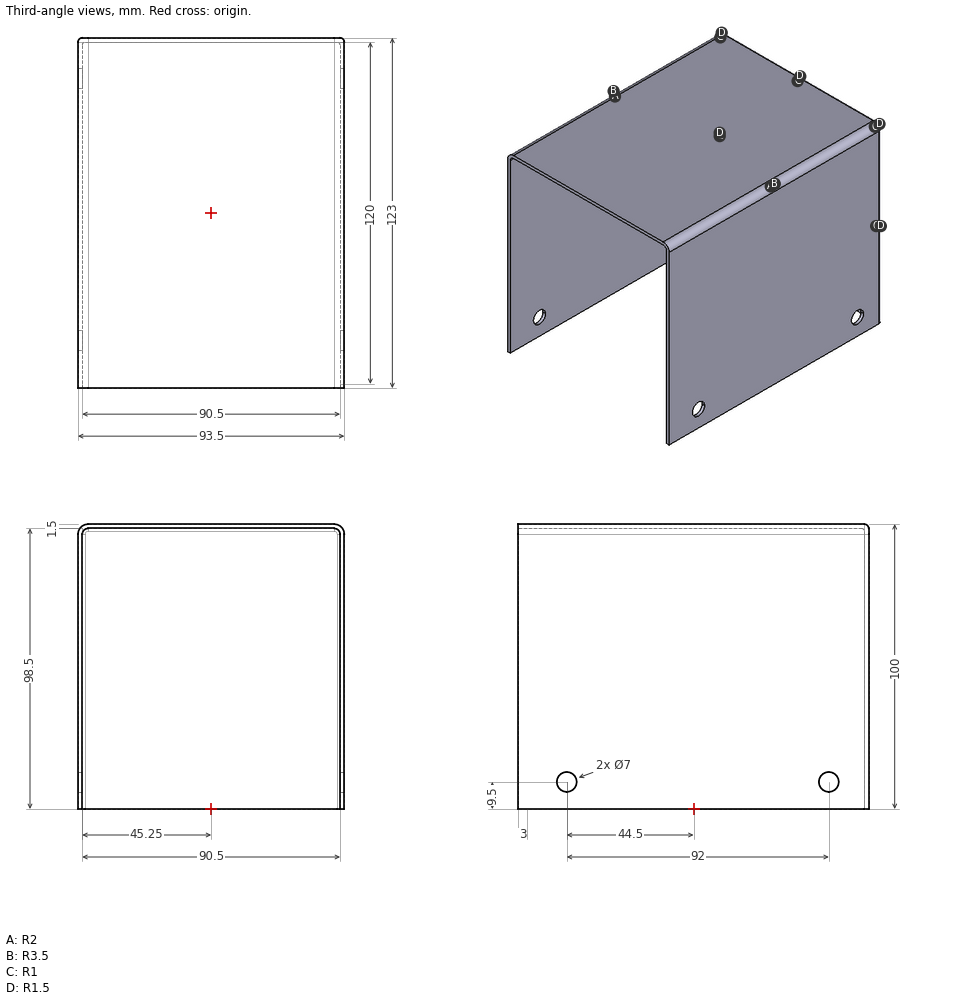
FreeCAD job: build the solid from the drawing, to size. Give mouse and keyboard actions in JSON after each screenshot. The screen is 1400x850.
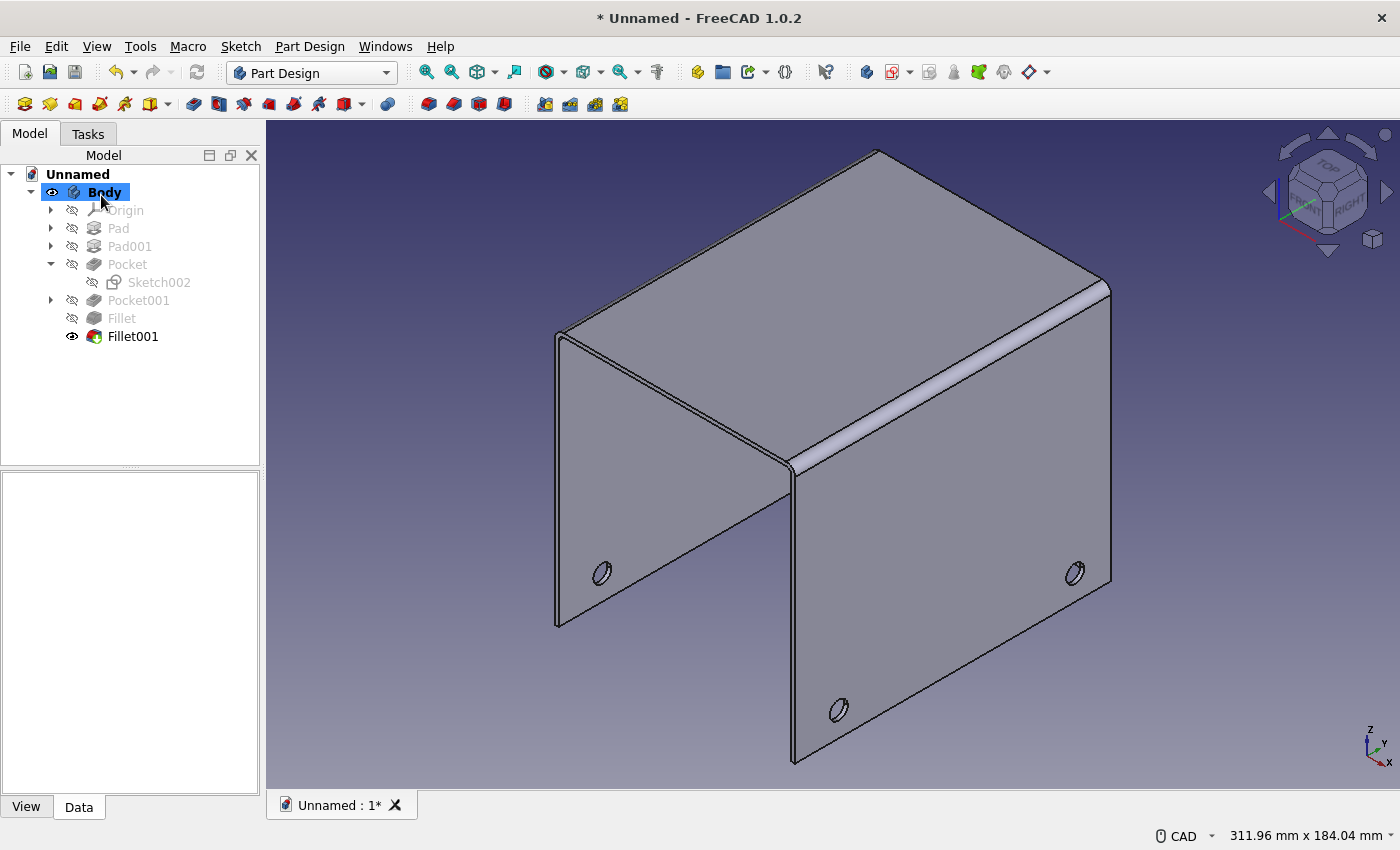
{"action": "key", "text": "2"}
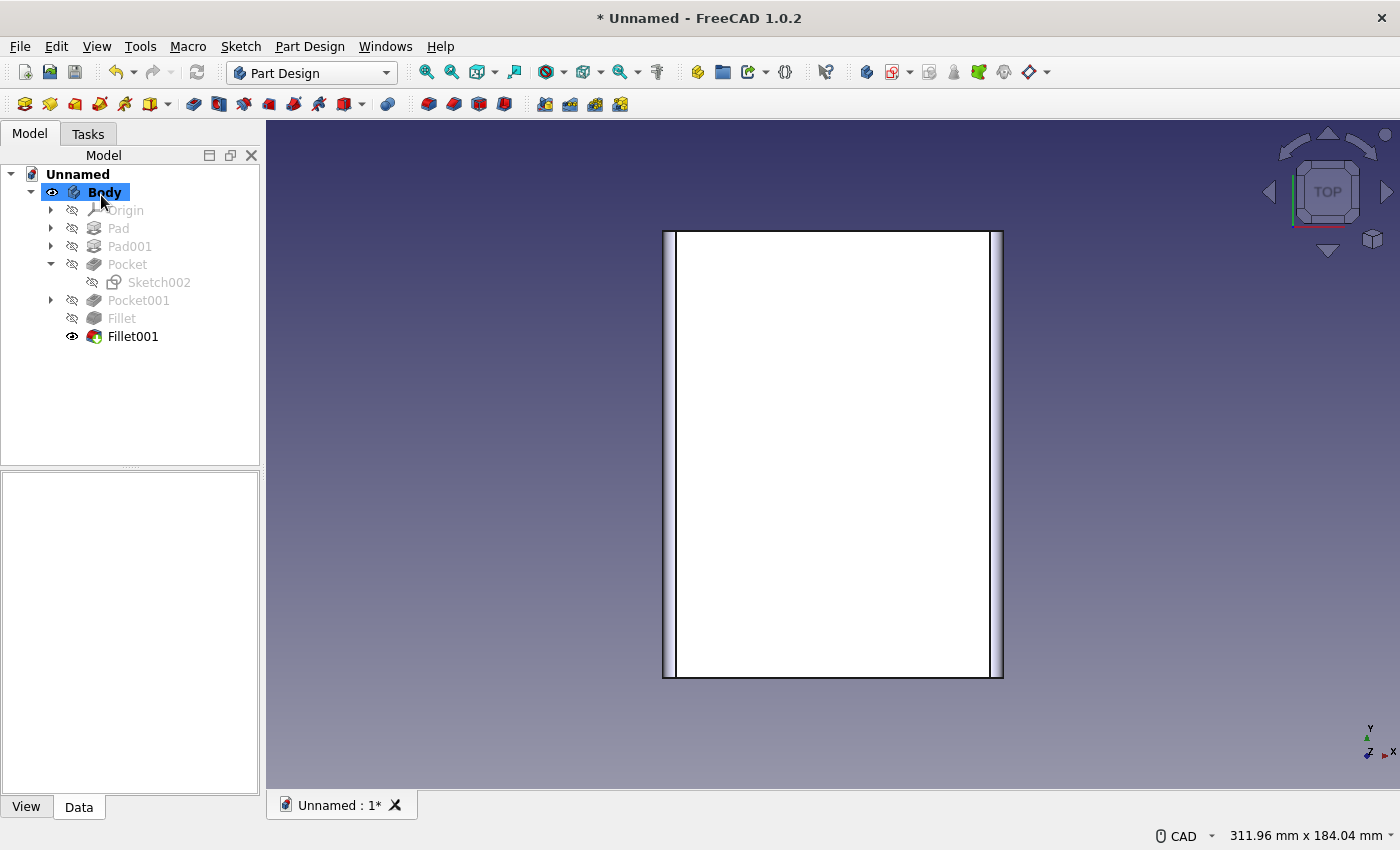
{"action": "key", "text": "1"}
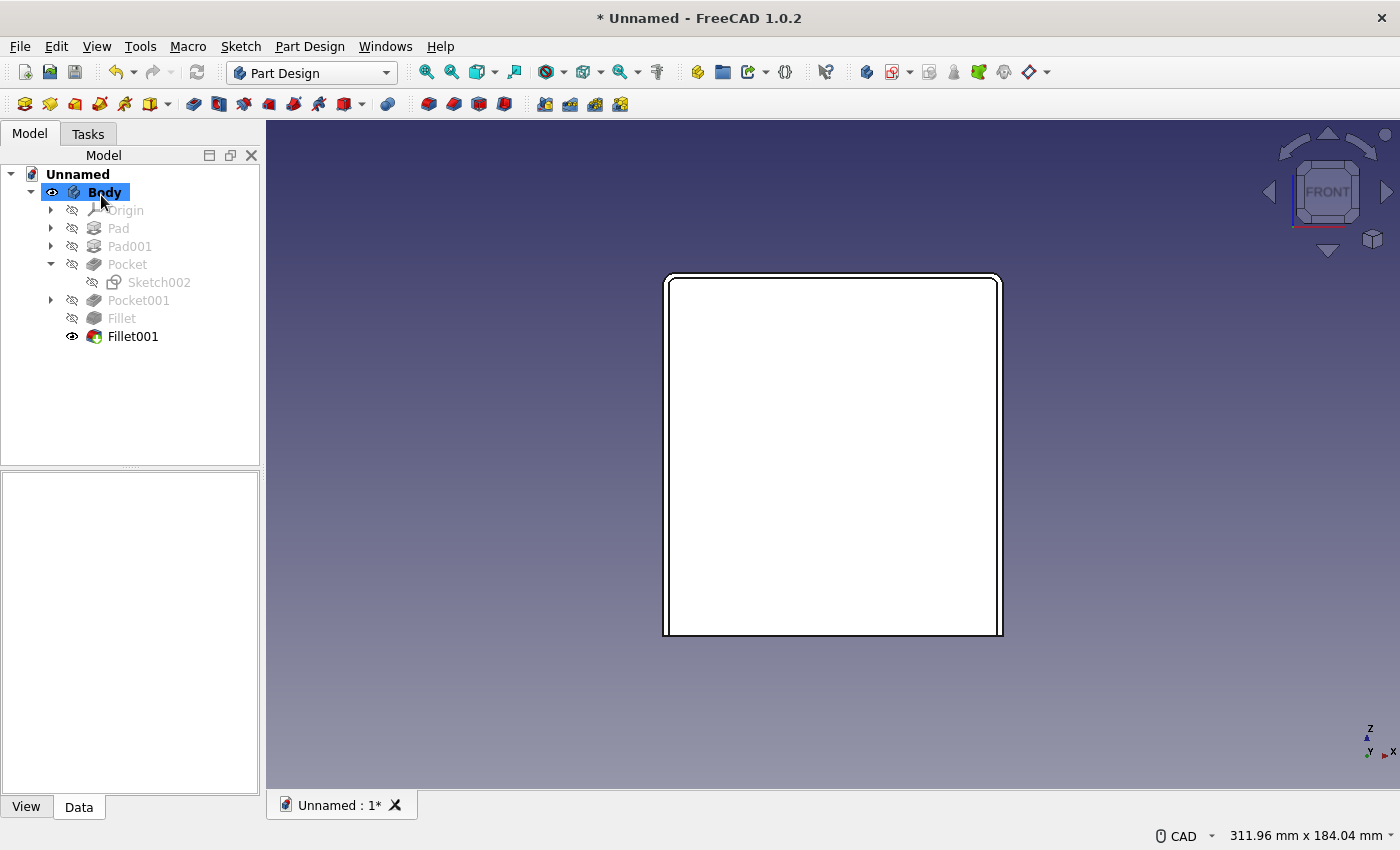
{"action": "key", "text": "3"}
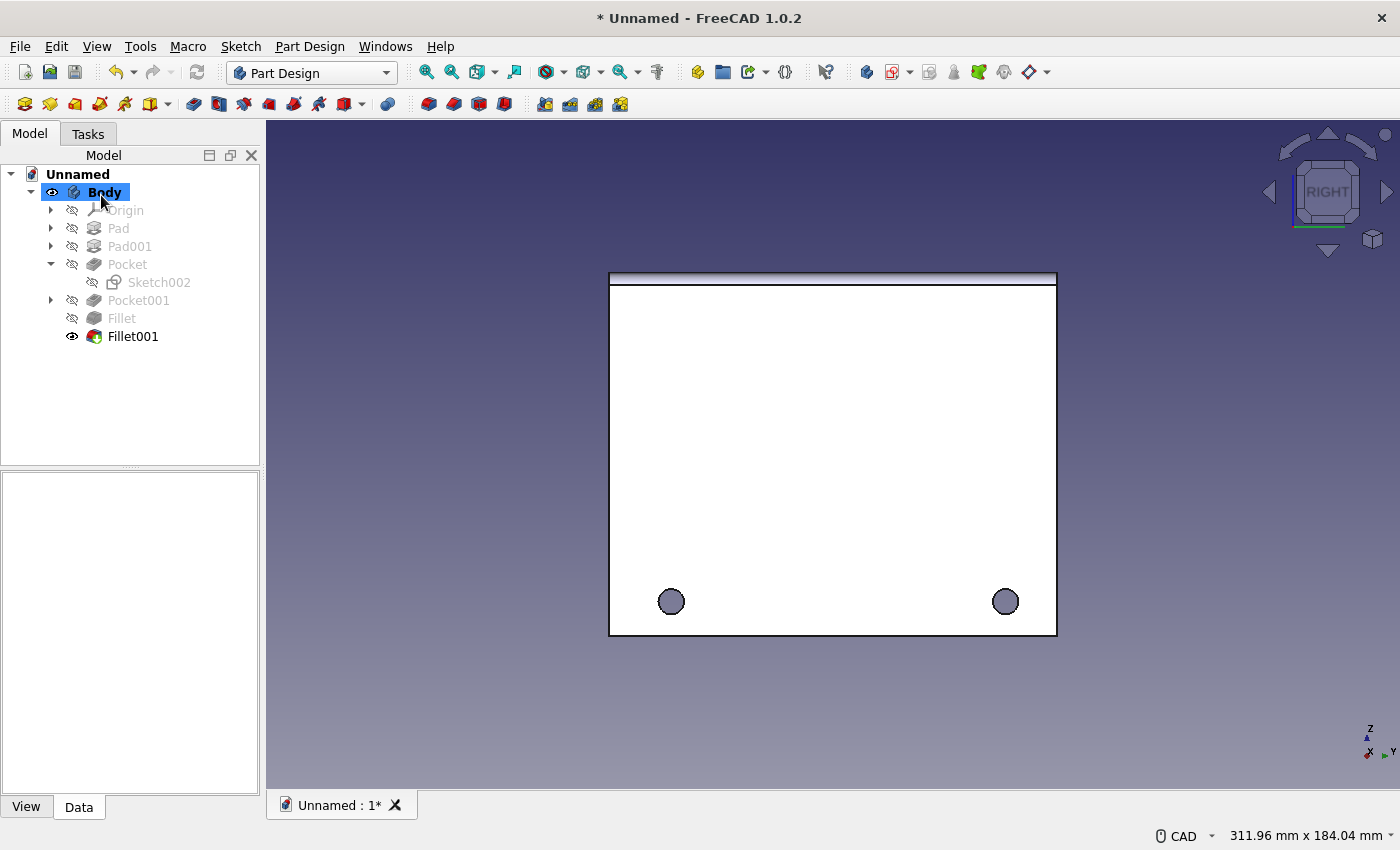
{"action": "key", "text": "5"}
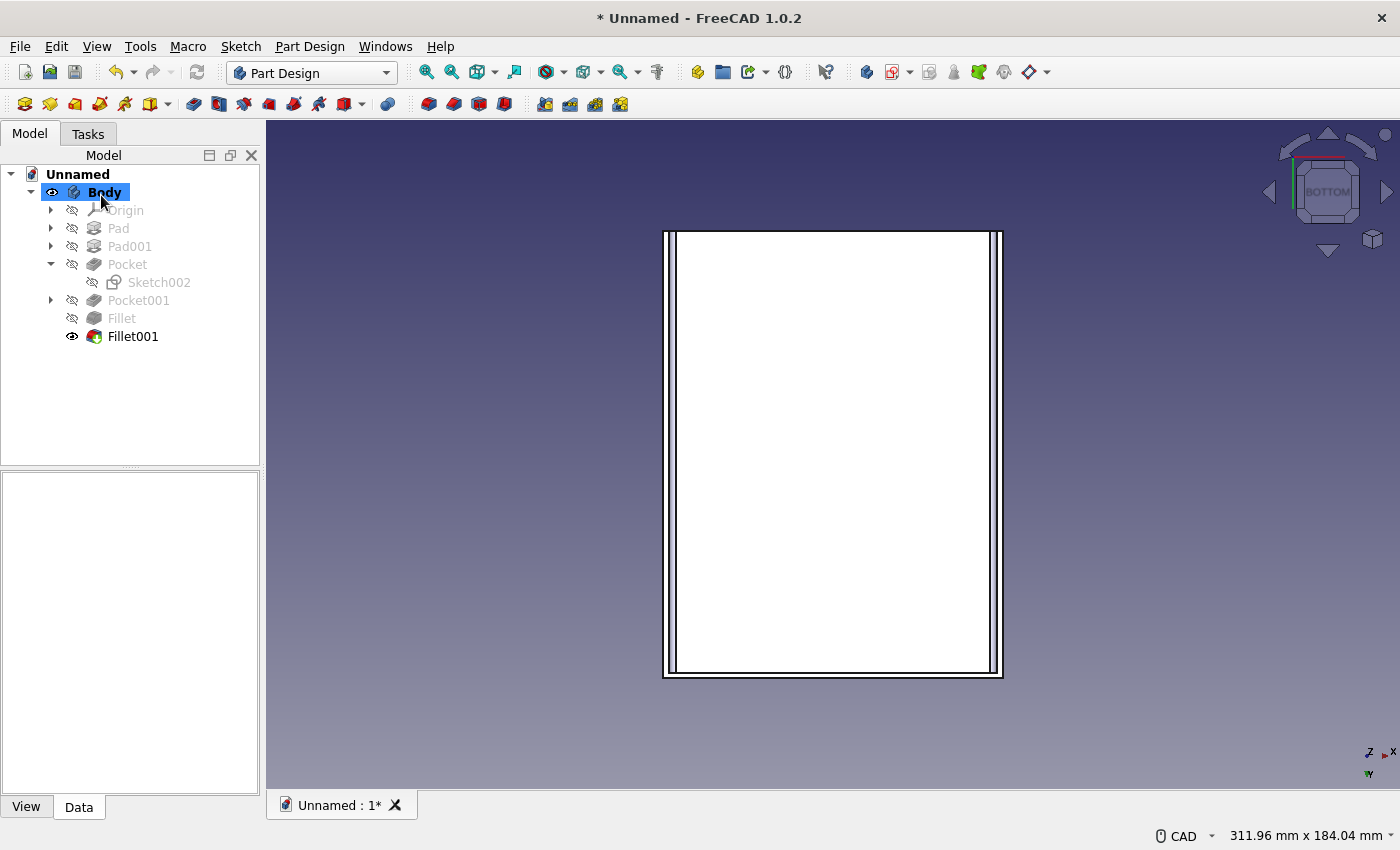
{"action": "key", "text": "4"}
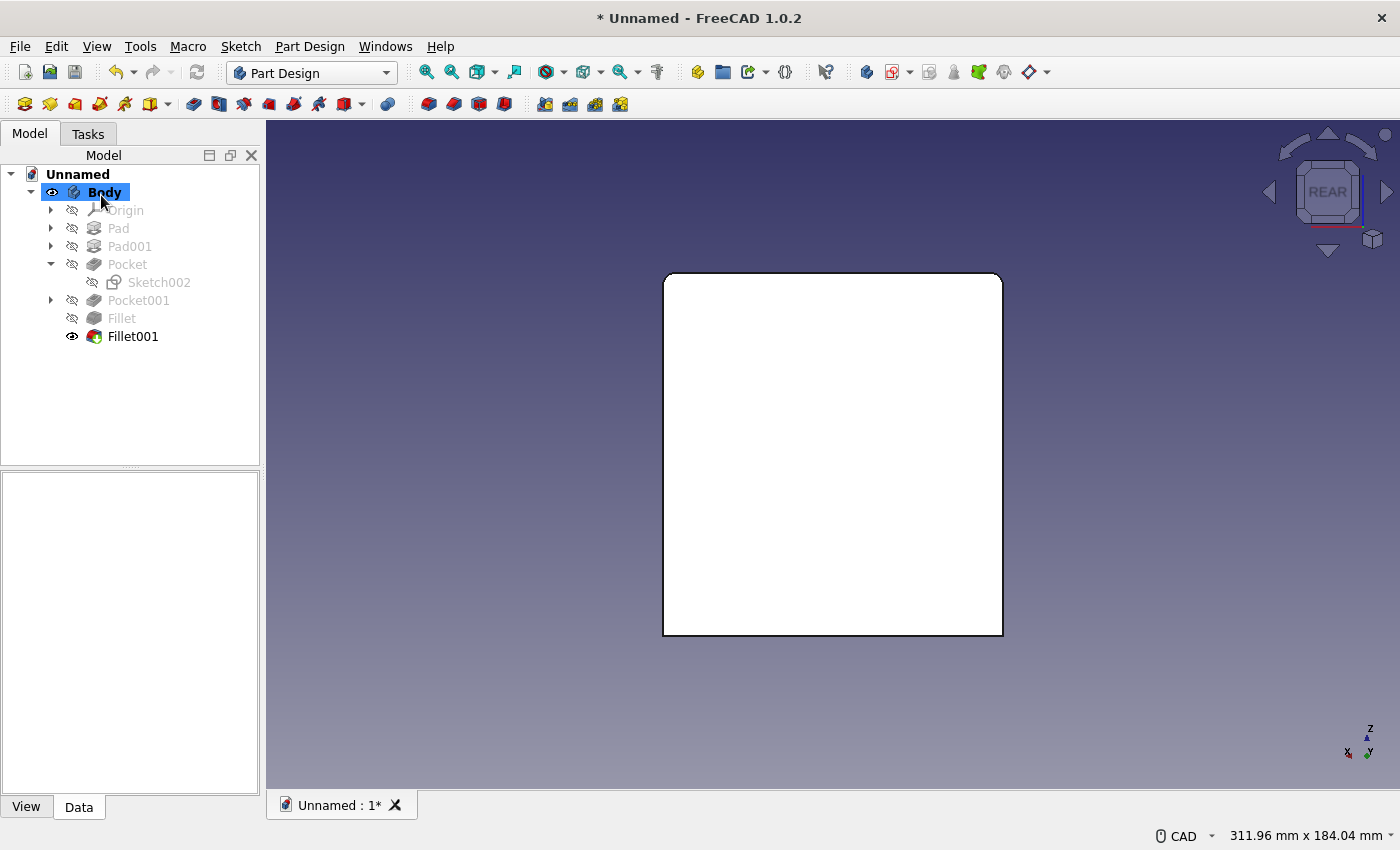
{"action": "key", "text": "6"}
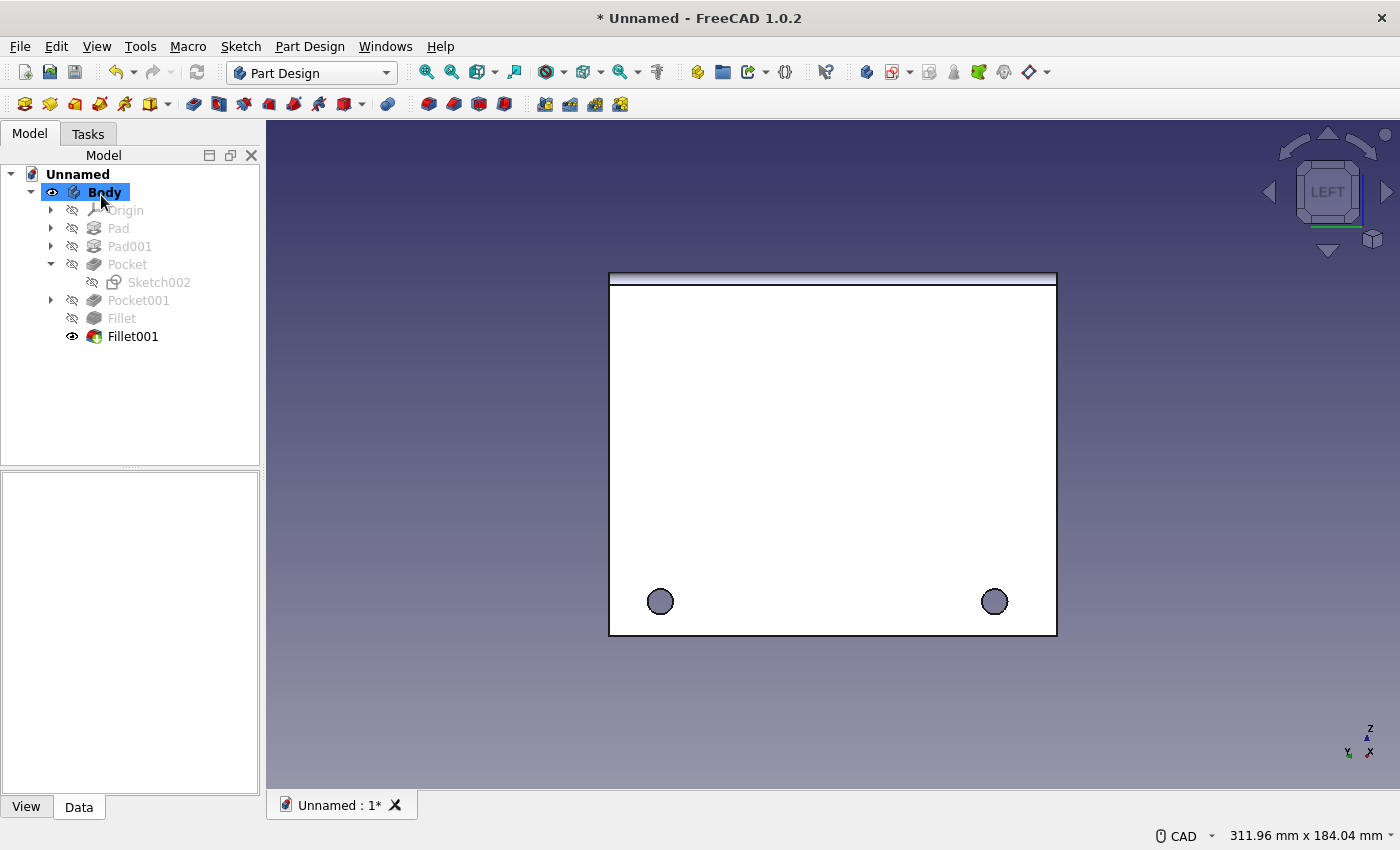
{"action": "key", "text": "v 3"}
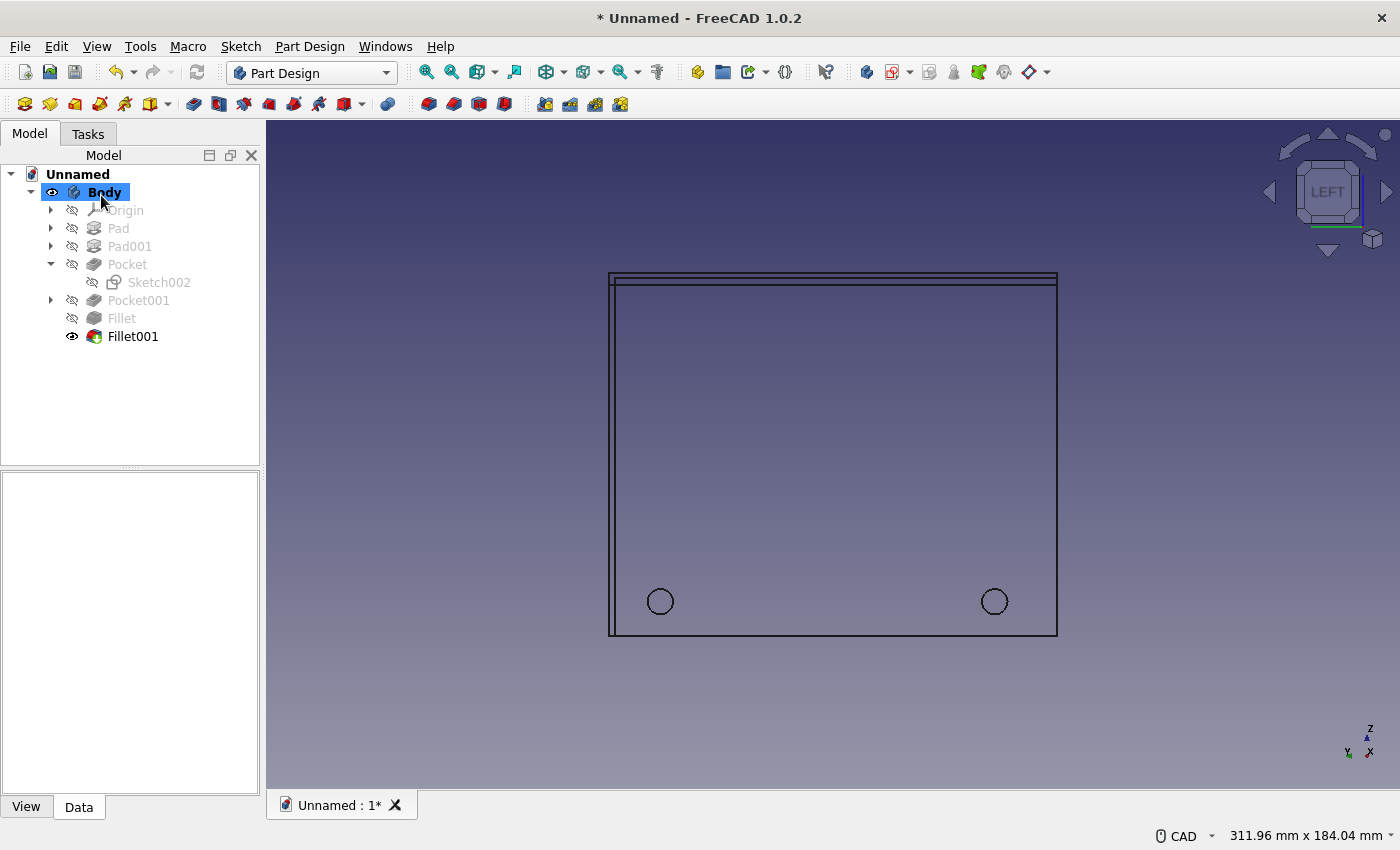
{"action": "key", "text": "0"}